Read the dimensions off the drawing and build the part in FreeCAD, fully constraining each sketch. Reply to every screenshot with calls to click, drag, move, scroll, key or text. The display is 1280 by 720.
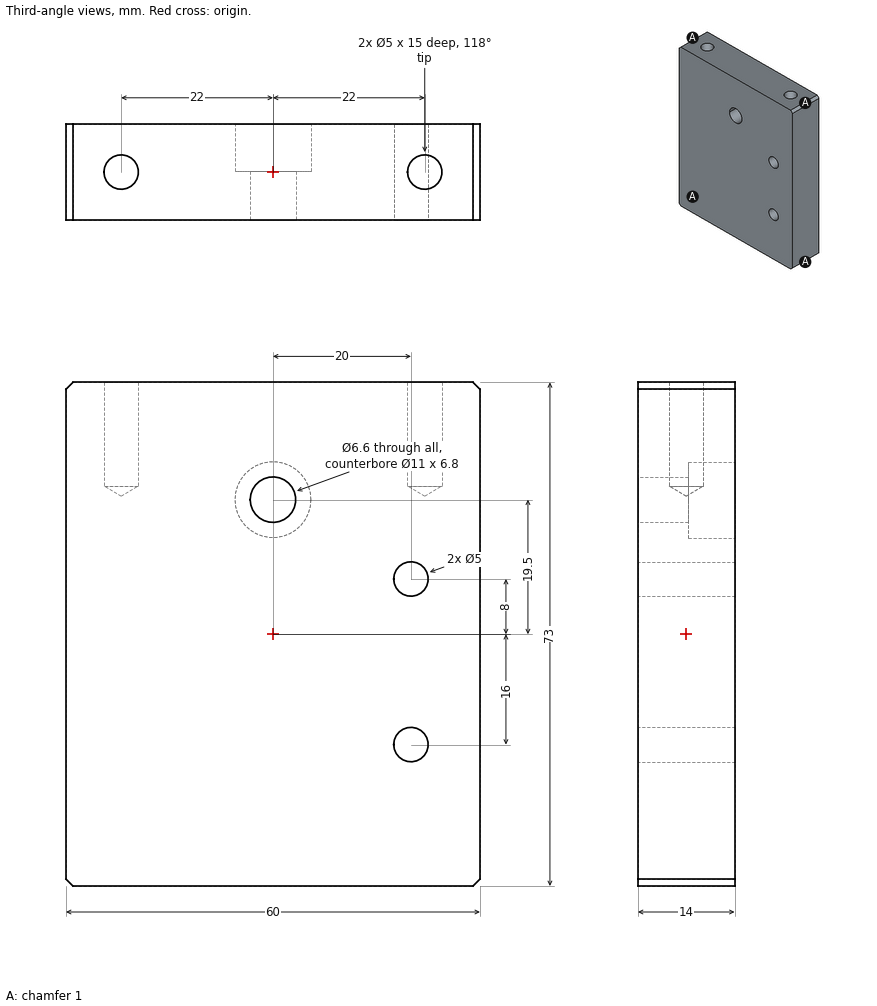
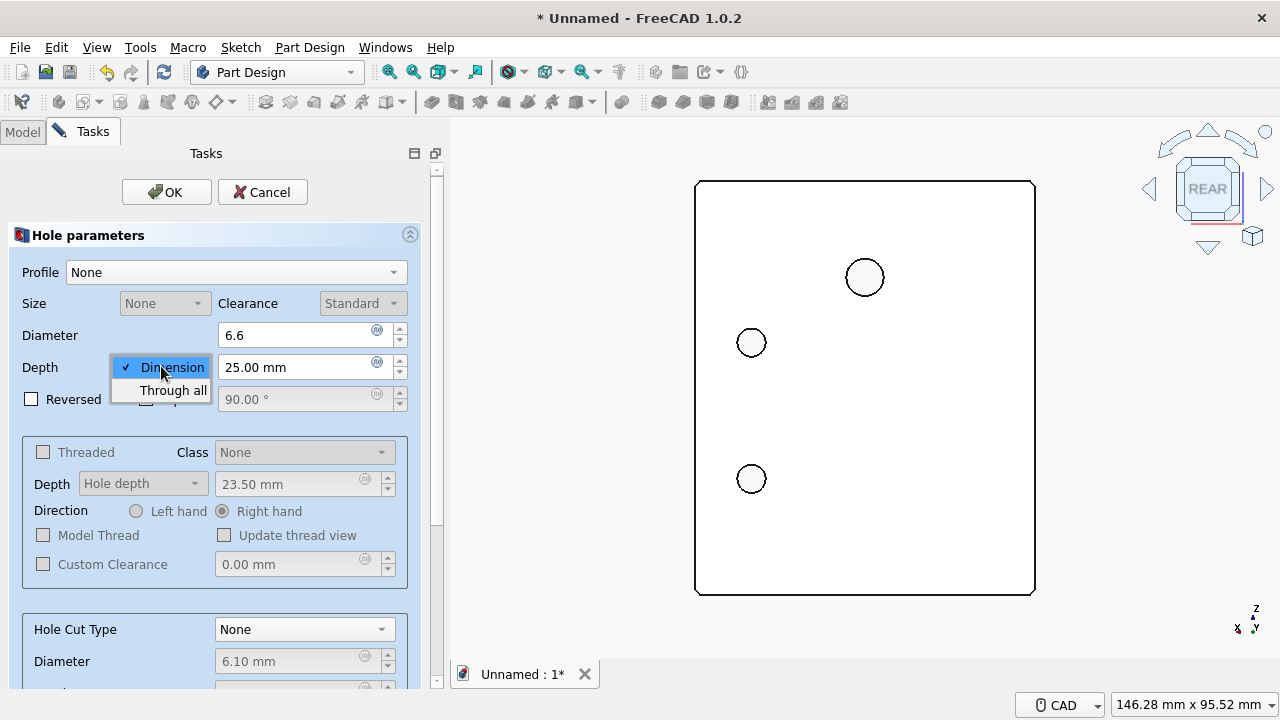
click(160, 390)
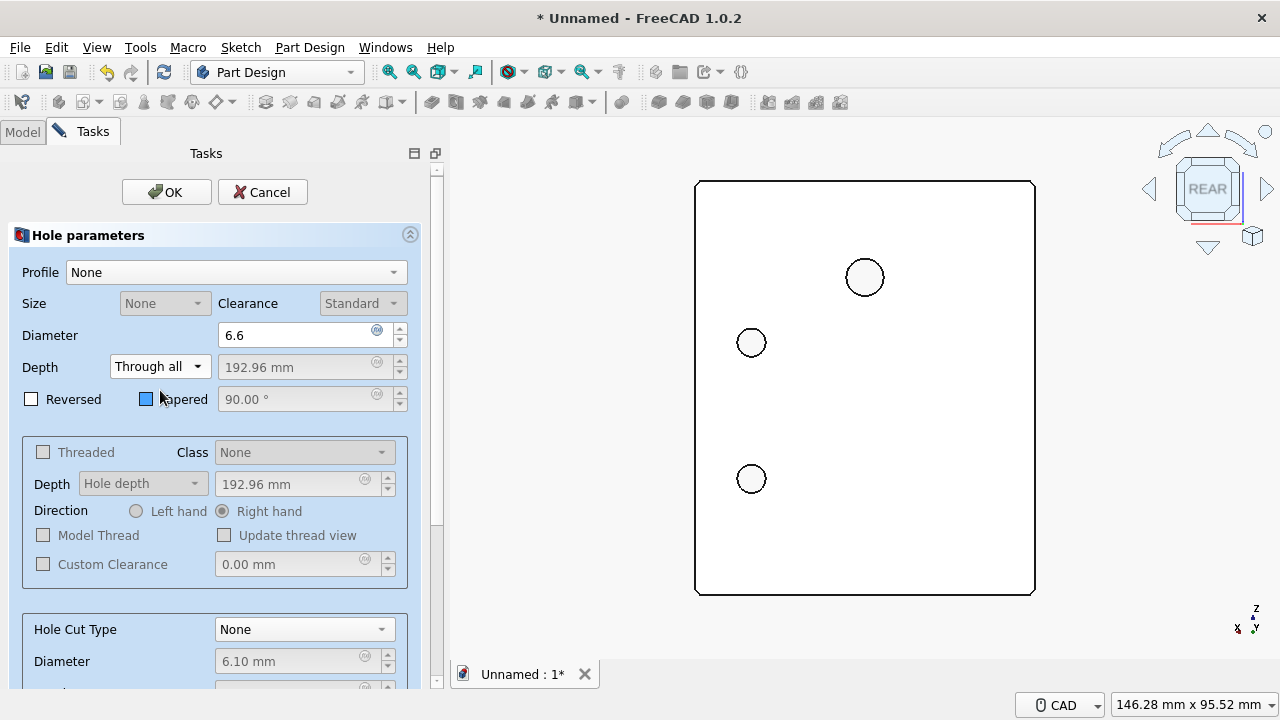
click(306, 630)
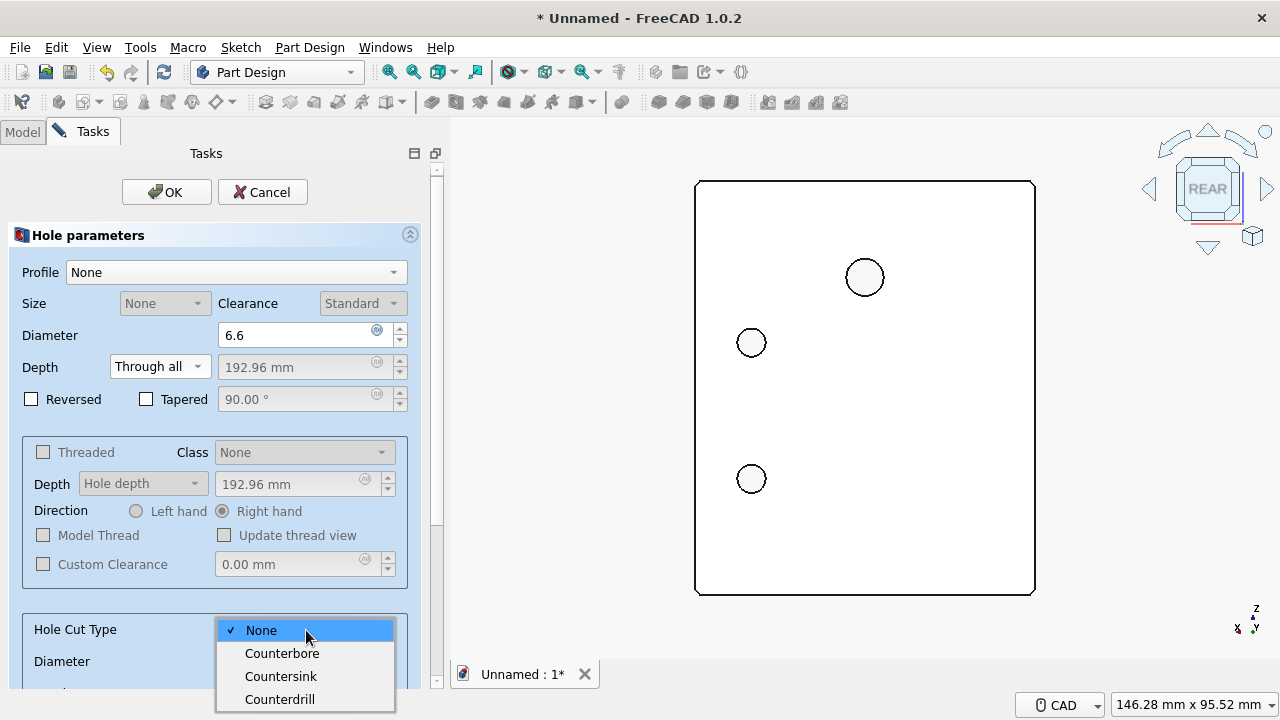
click(304, 654)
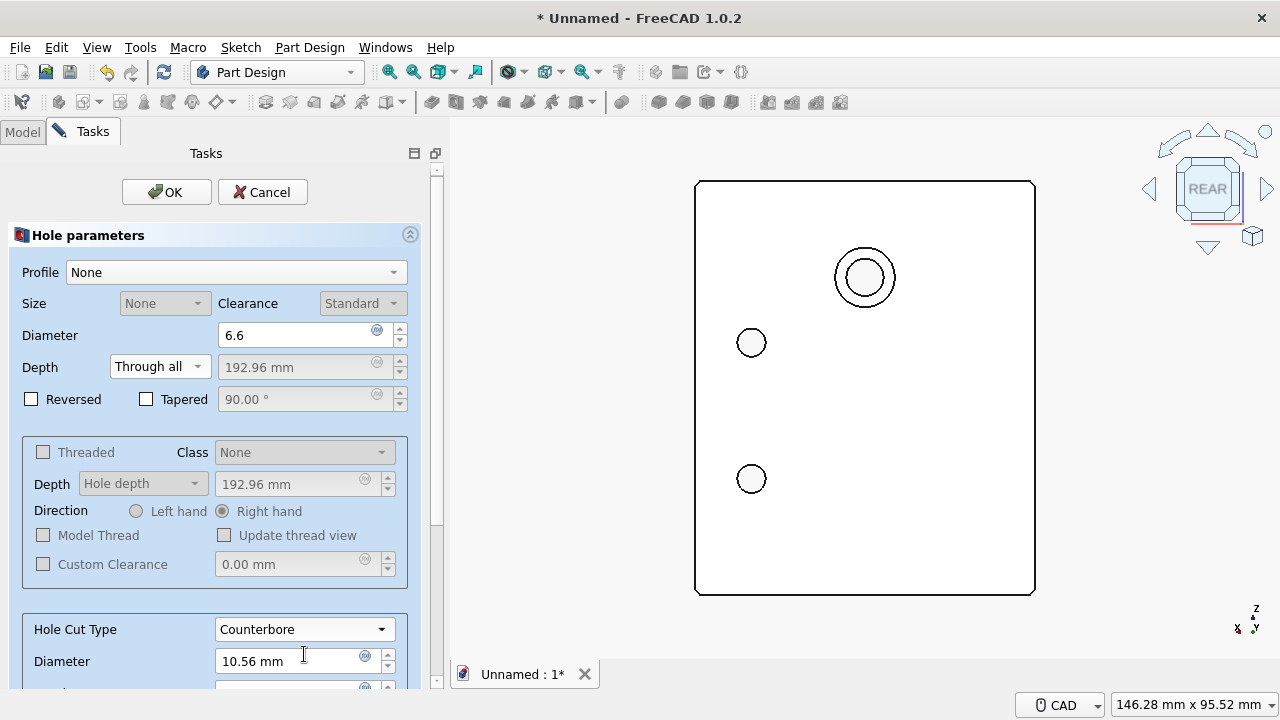
triple_click(298, 661)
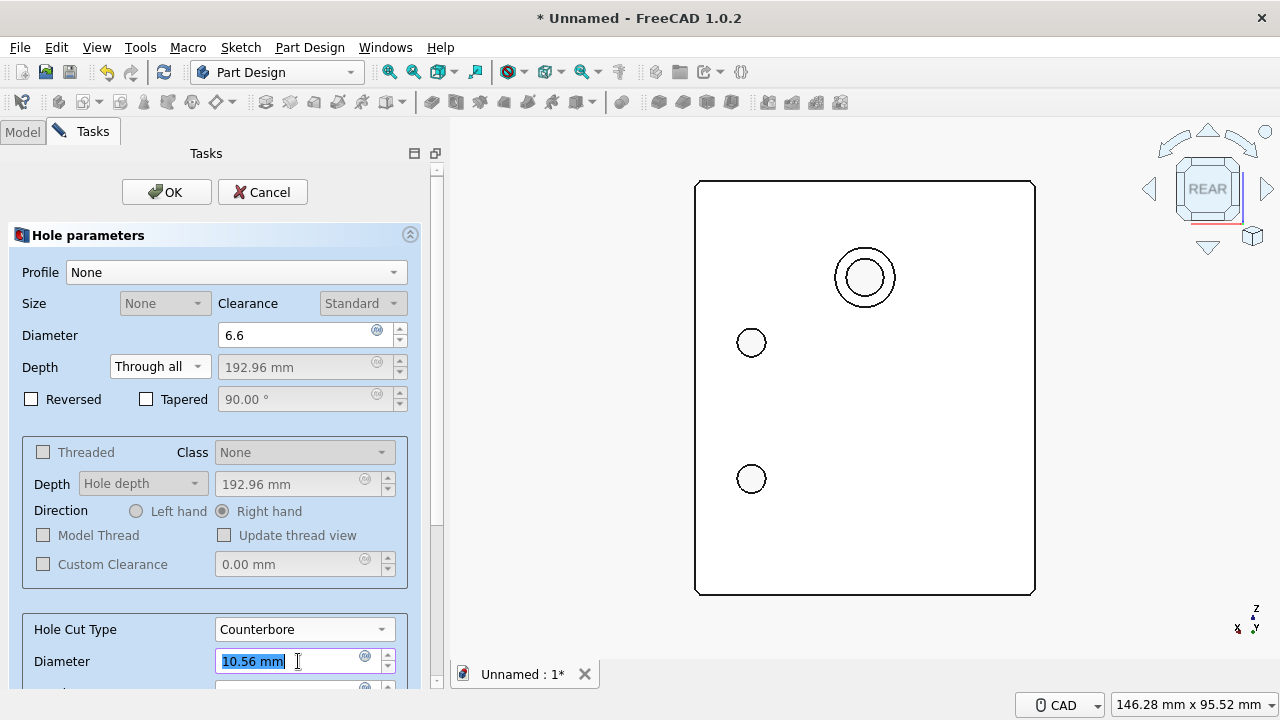
text(11)
key(Tab)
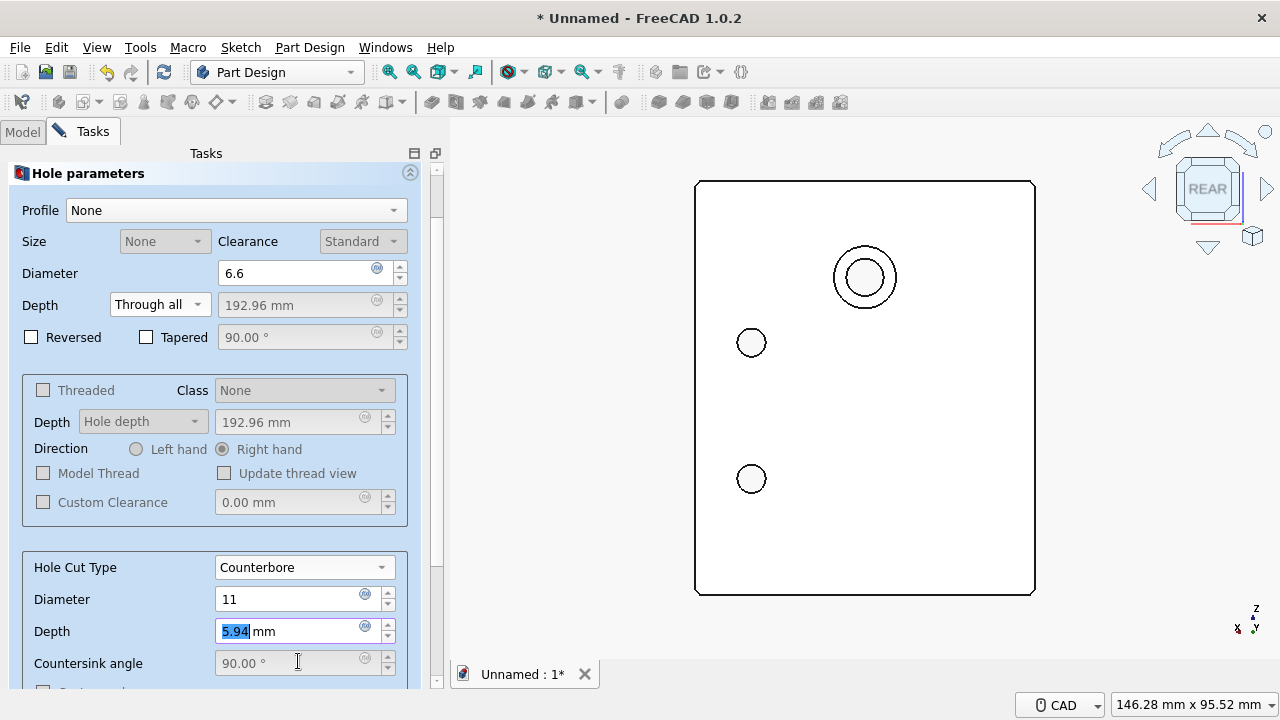
text(6.8)
key(Tab)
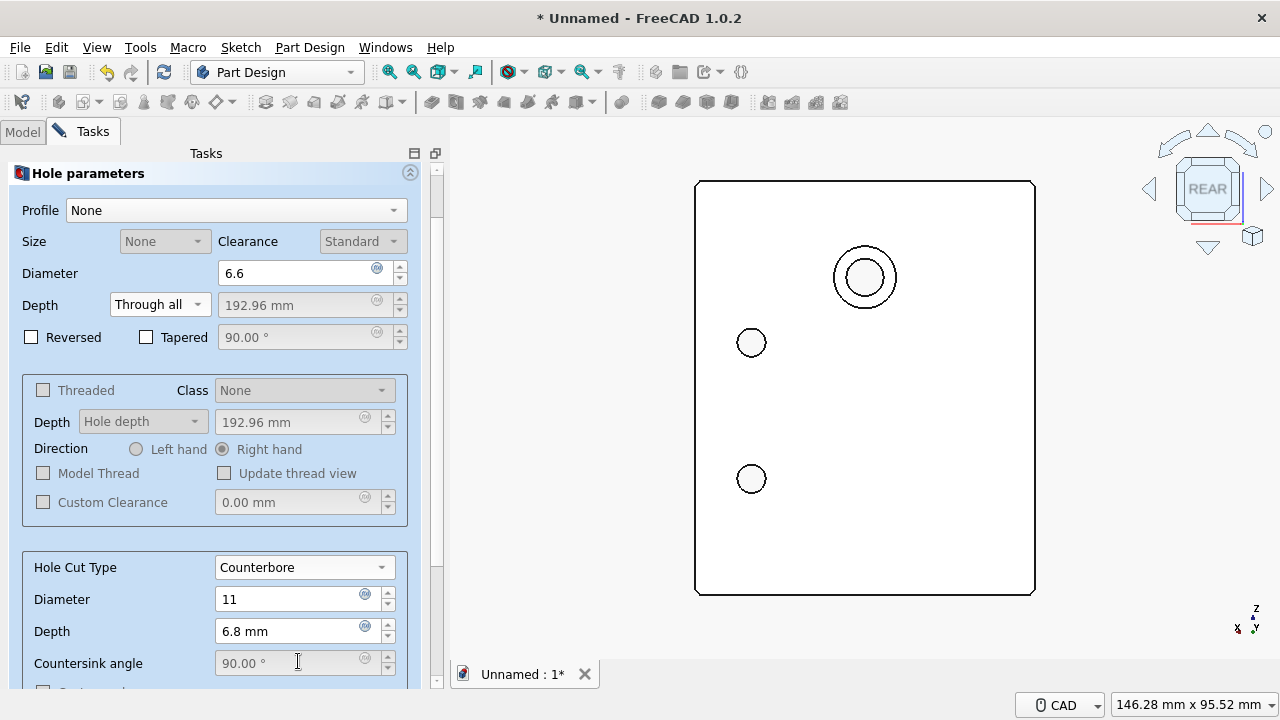
scroll(437, 426, up, 2)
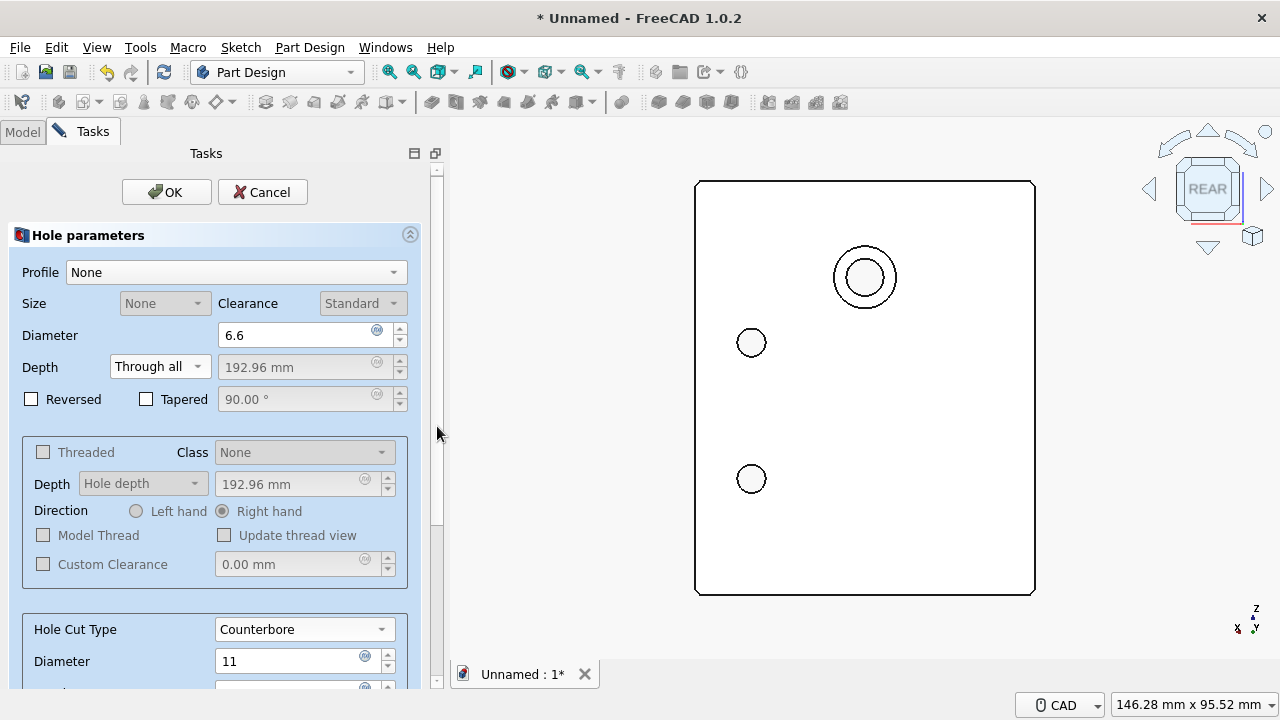
click(167, 192)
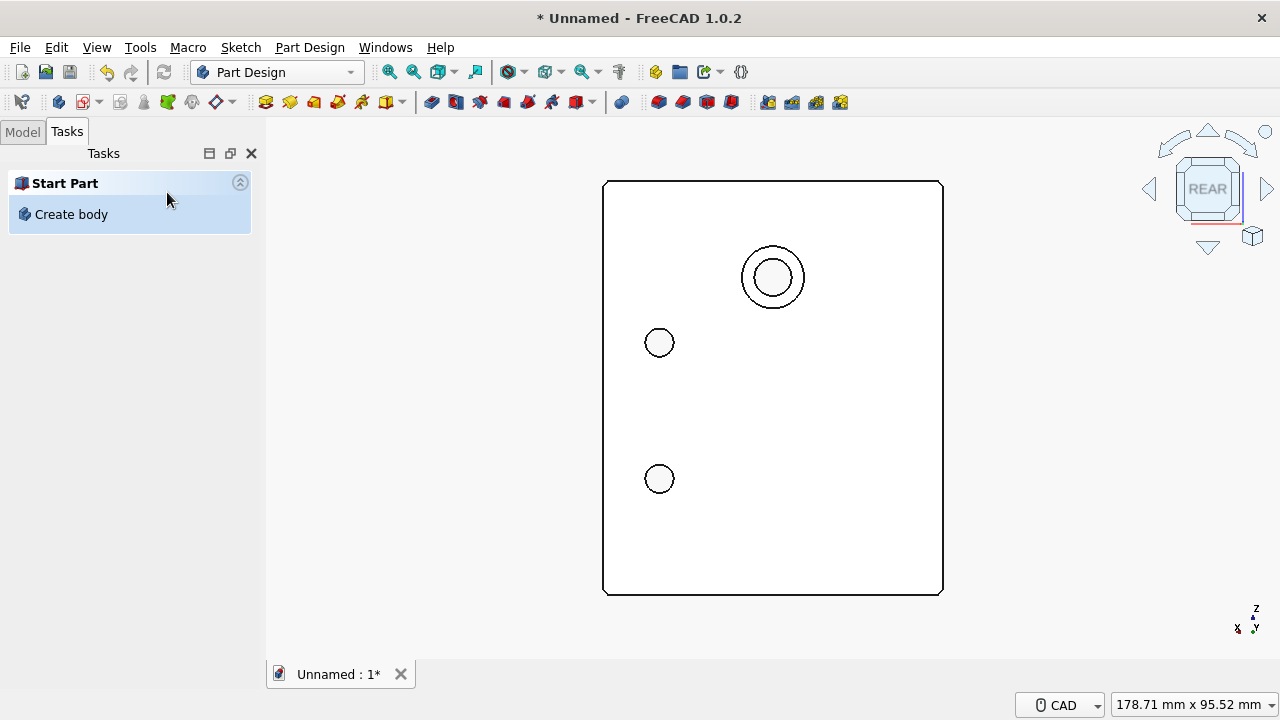
key(0)